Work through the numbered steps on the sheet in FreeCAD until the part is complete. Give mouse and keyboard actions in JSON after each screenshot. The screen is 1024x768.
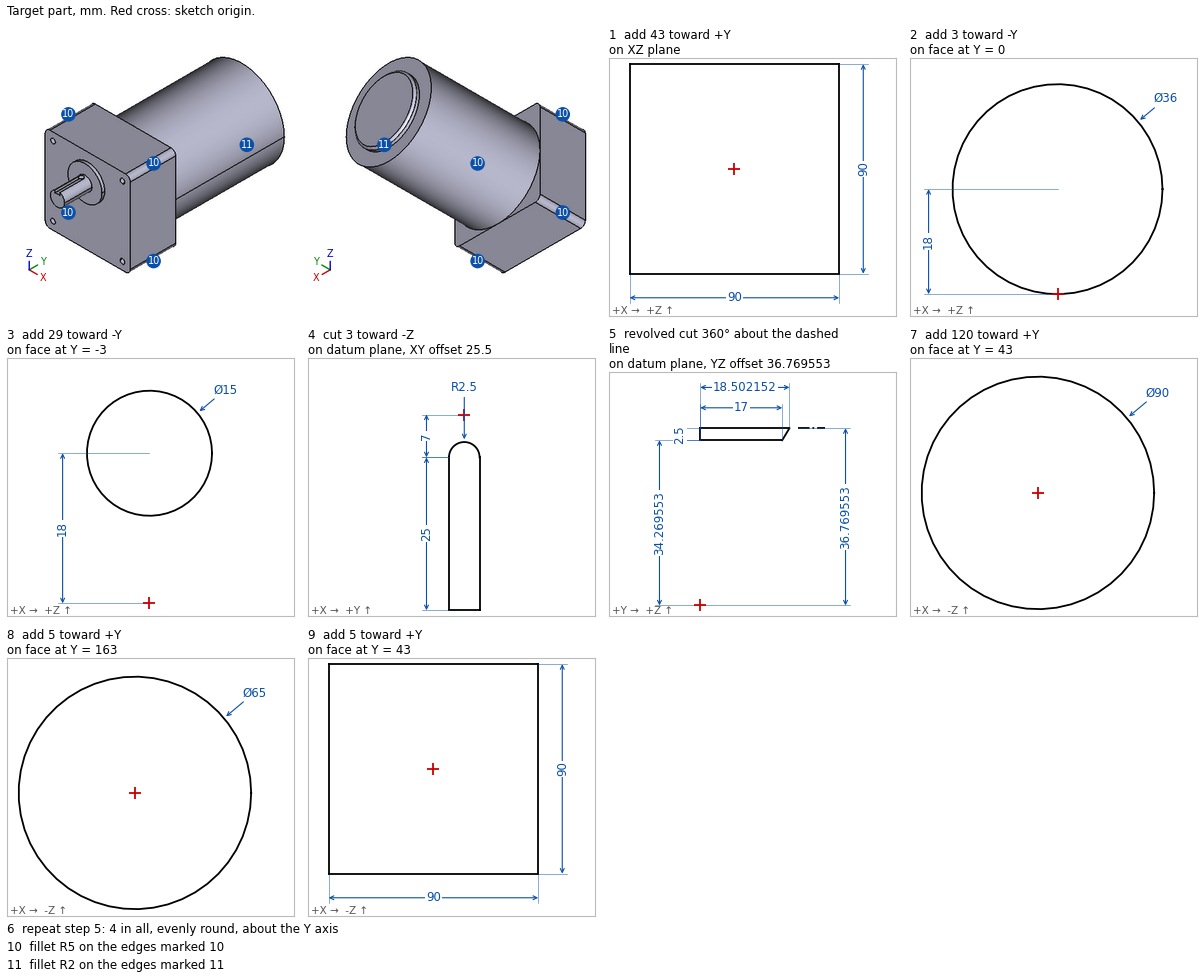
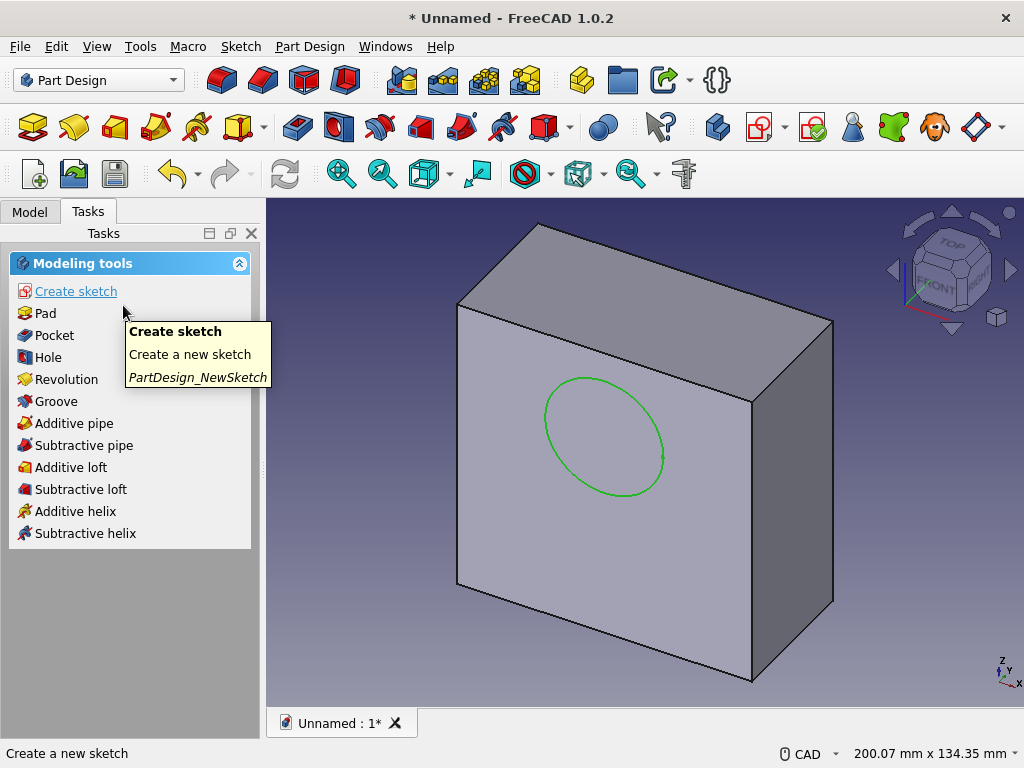
{"action": "left_click", "coordinate": [33, 128]}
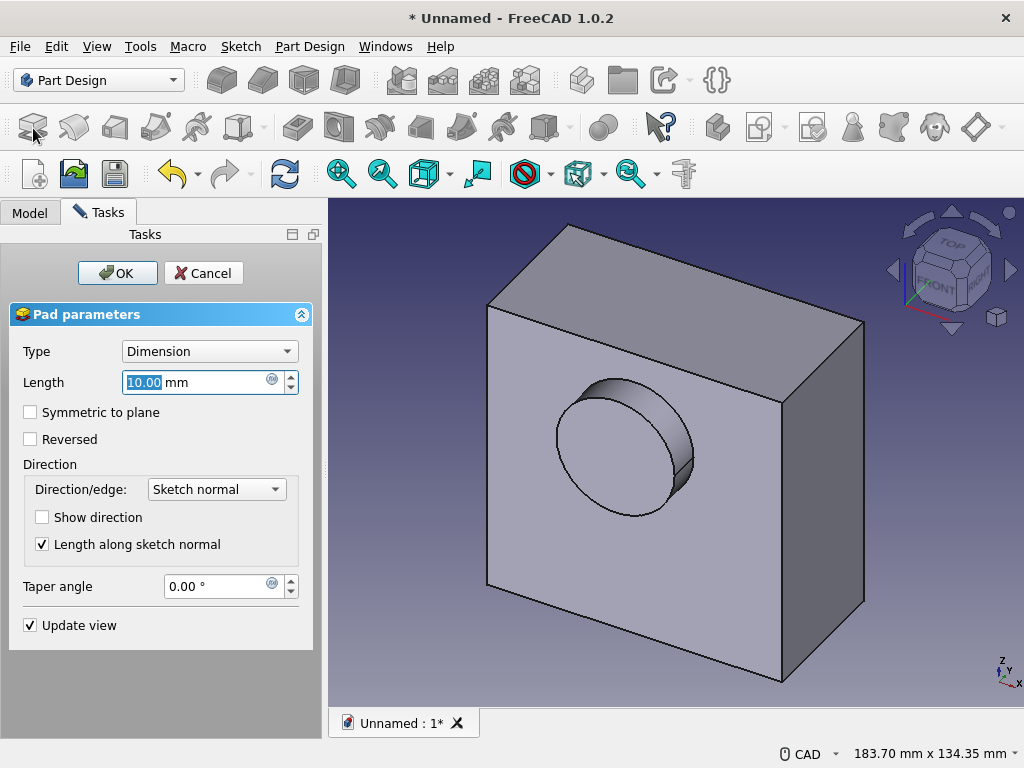
{"action": "type", "text": "3"}
{"action": "key", "text": "Tab"}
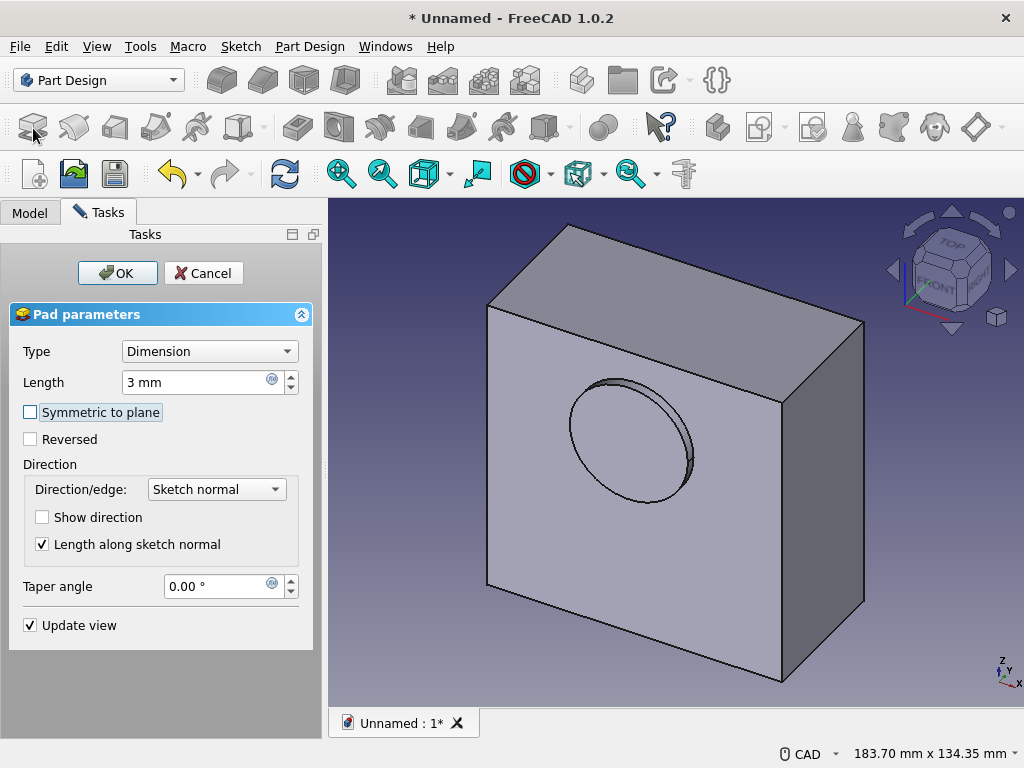
{"action": "left_click", "coordinate": [118, 273]}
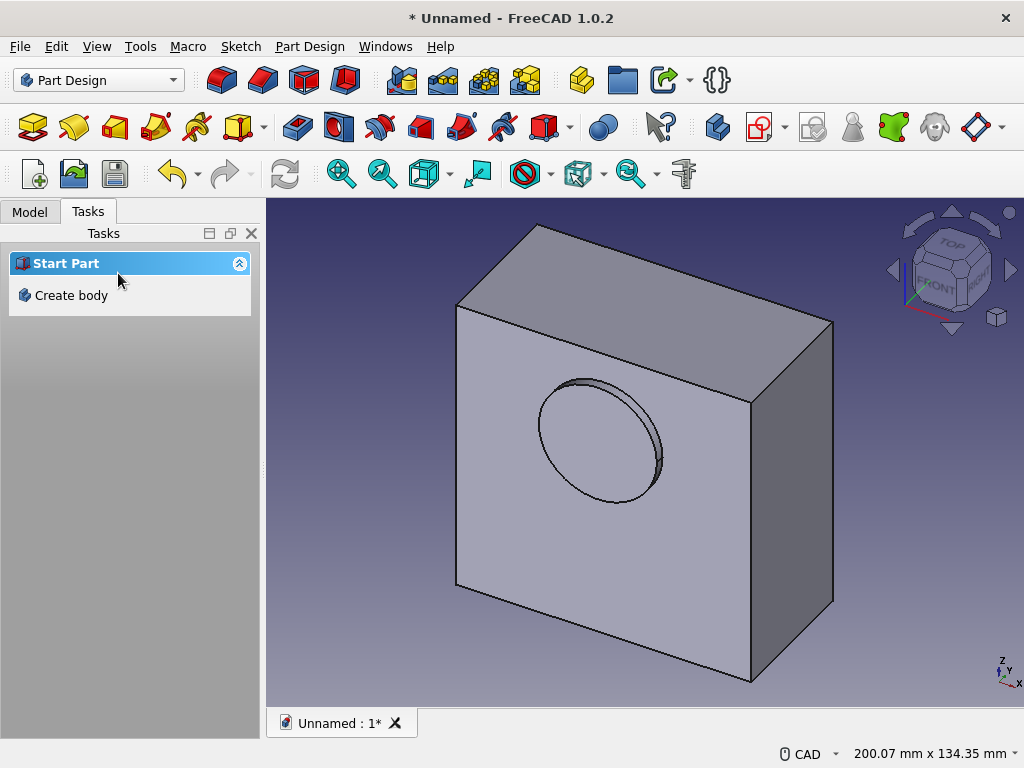
{"action": "left_click", "coordinate": [598, 443]}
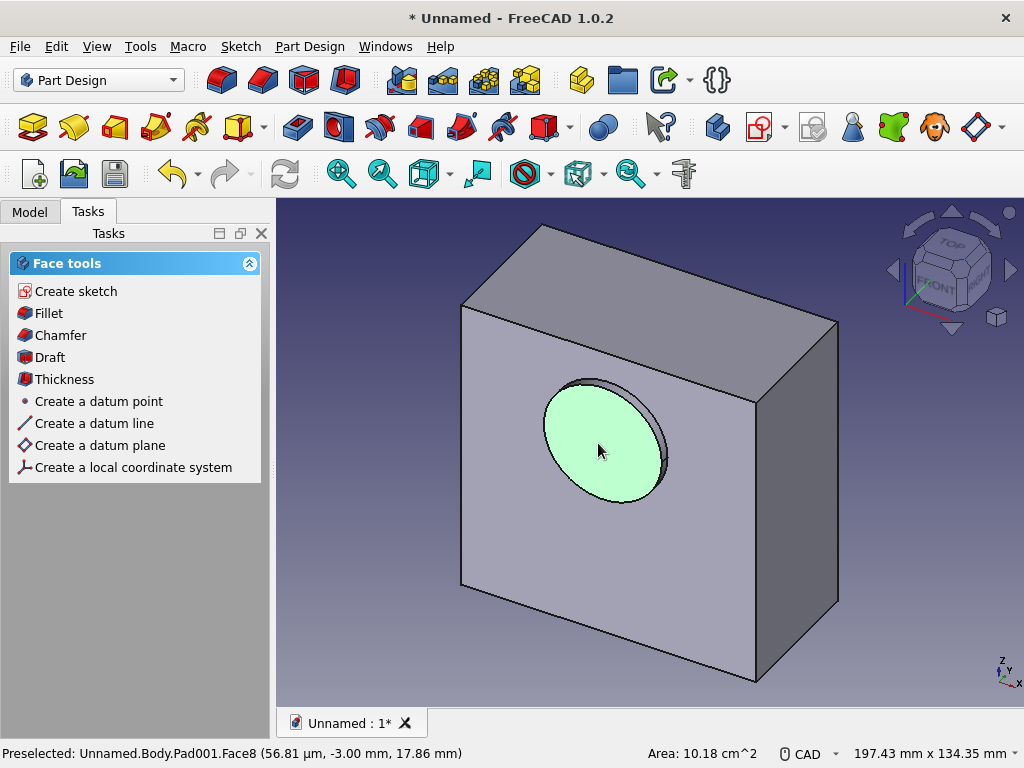
{"action": "left_click", "coordinate": [758, 128]}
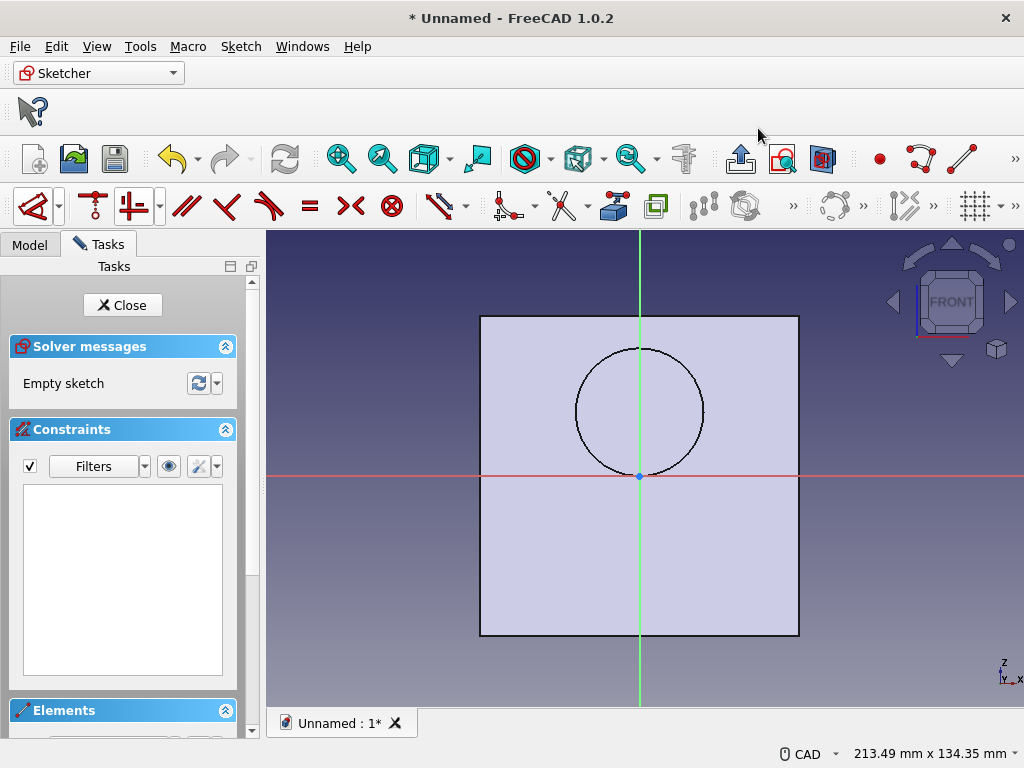
{"action": "scroll", "coordinate": [667, 415], "scroll_direction": "up", "scroll_amount": 6}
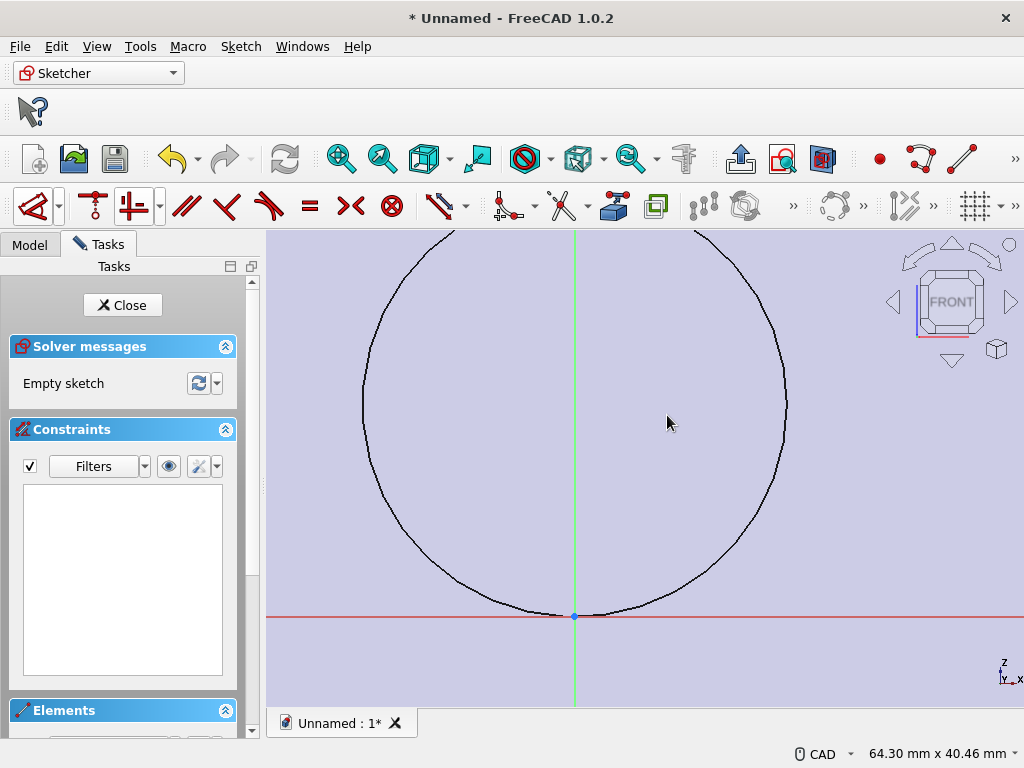
{"action": "key", "text": "g c"}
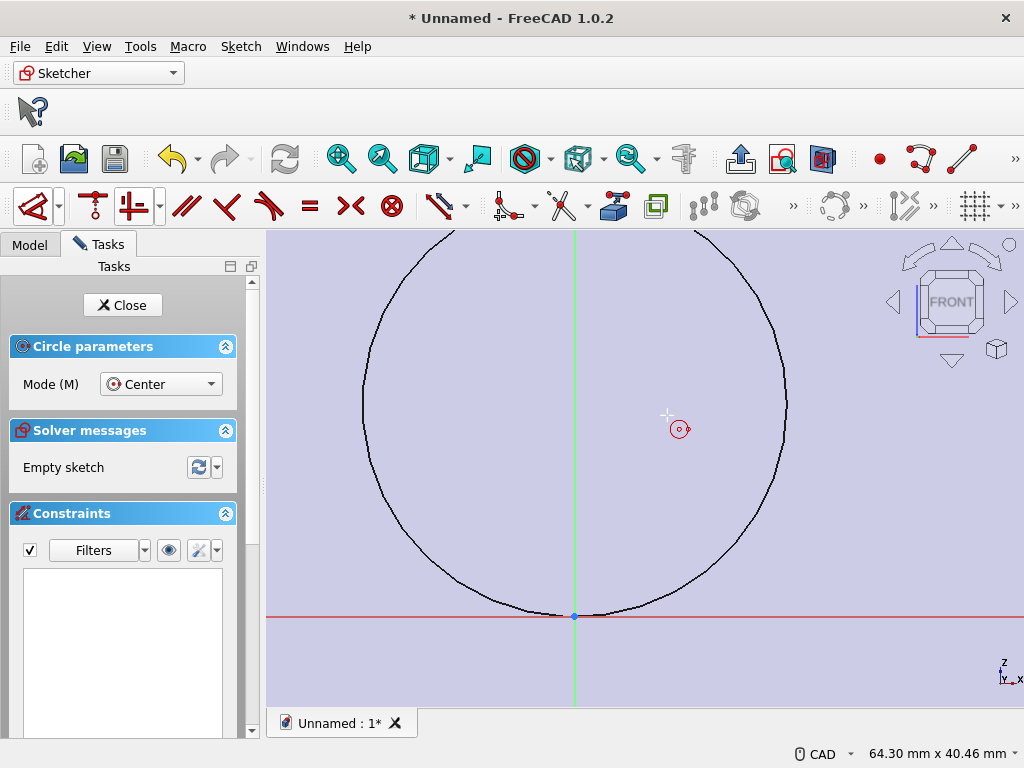
{"action": "left_click", "coordinate": [575, 405]}
{"action": "mouse_move", "coordinate": [637, 342]}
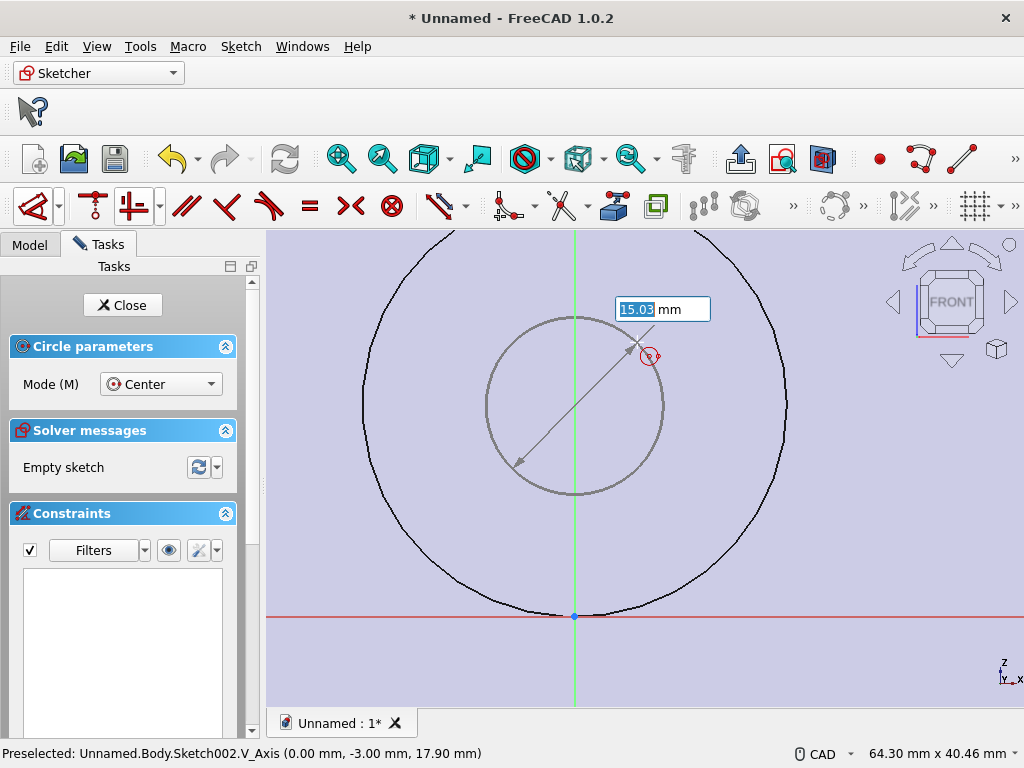
{"action": "type", "text": "15"}
{"action": "key", "text": "Return"}
{"action": "key", "text": "Escape"}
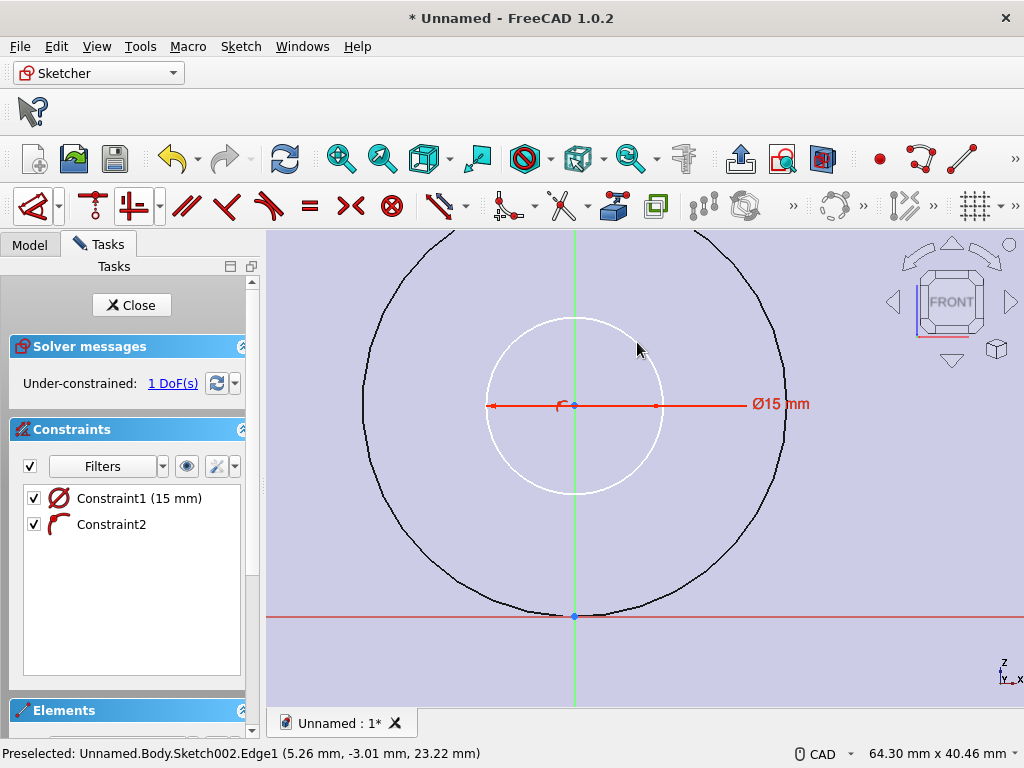
{"action": "left_click", "coordinate": [575, 406]}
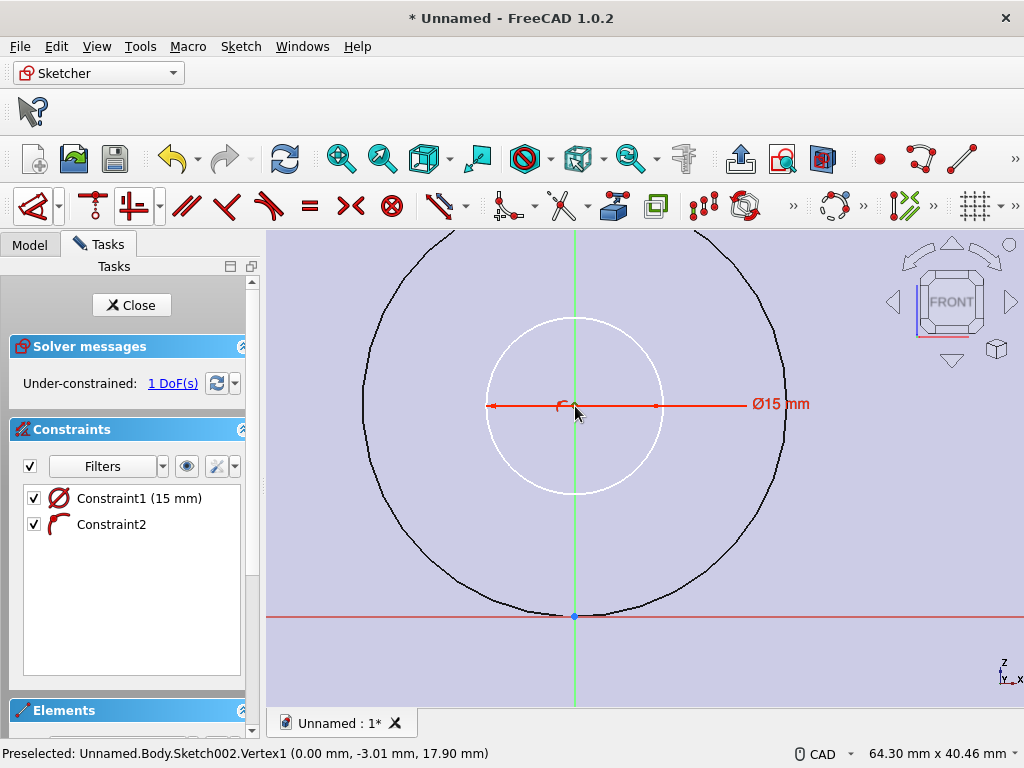
{"action": "key", "text": "i"}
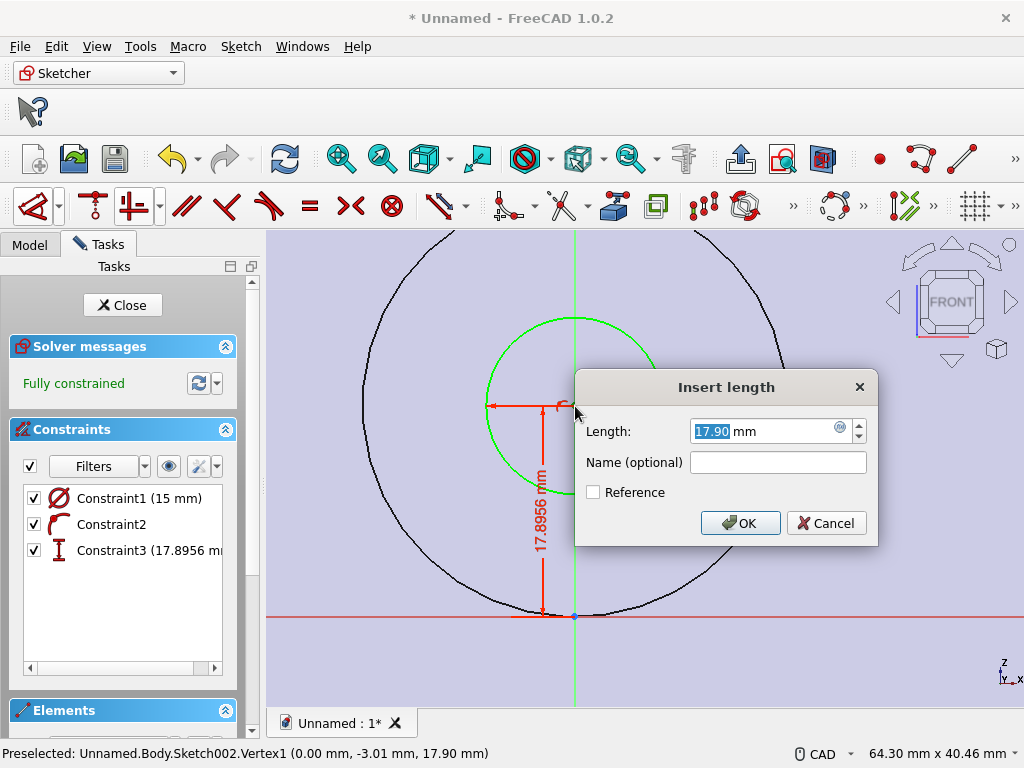
{"action": "type", "text": "18"}
{"action": "key", "text": "Return"}